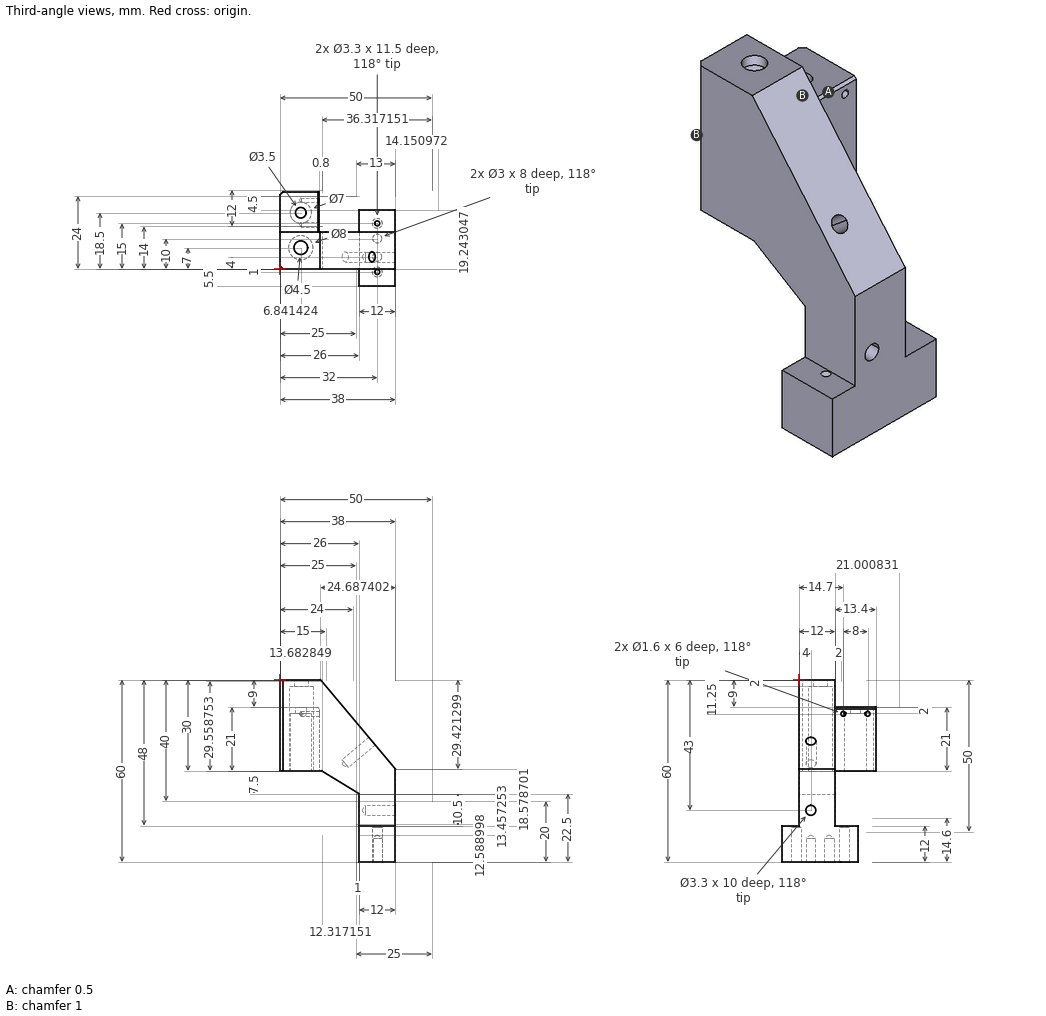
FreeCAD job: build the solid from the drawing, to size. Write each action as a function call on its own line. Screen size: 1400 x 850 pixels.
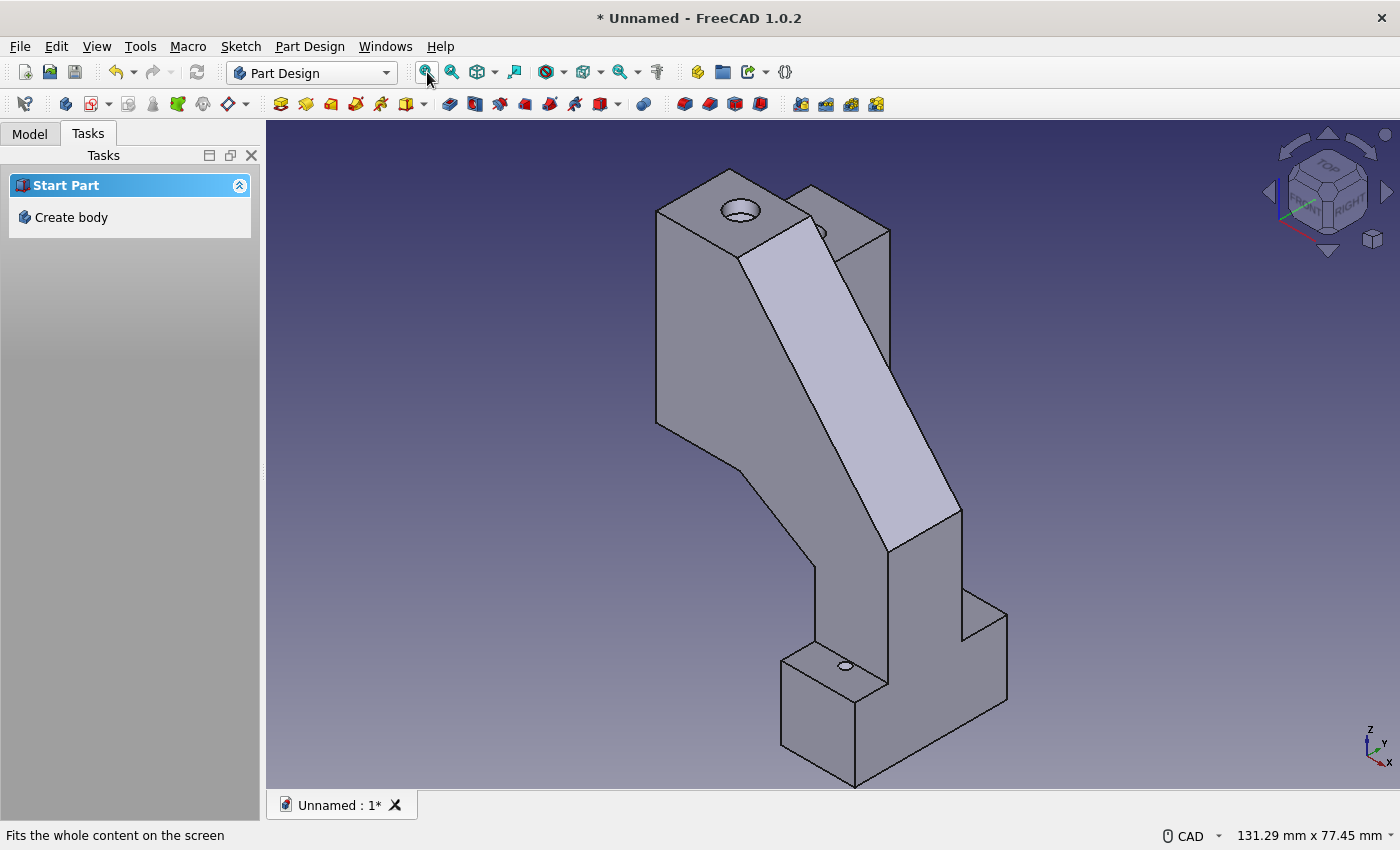
key(3)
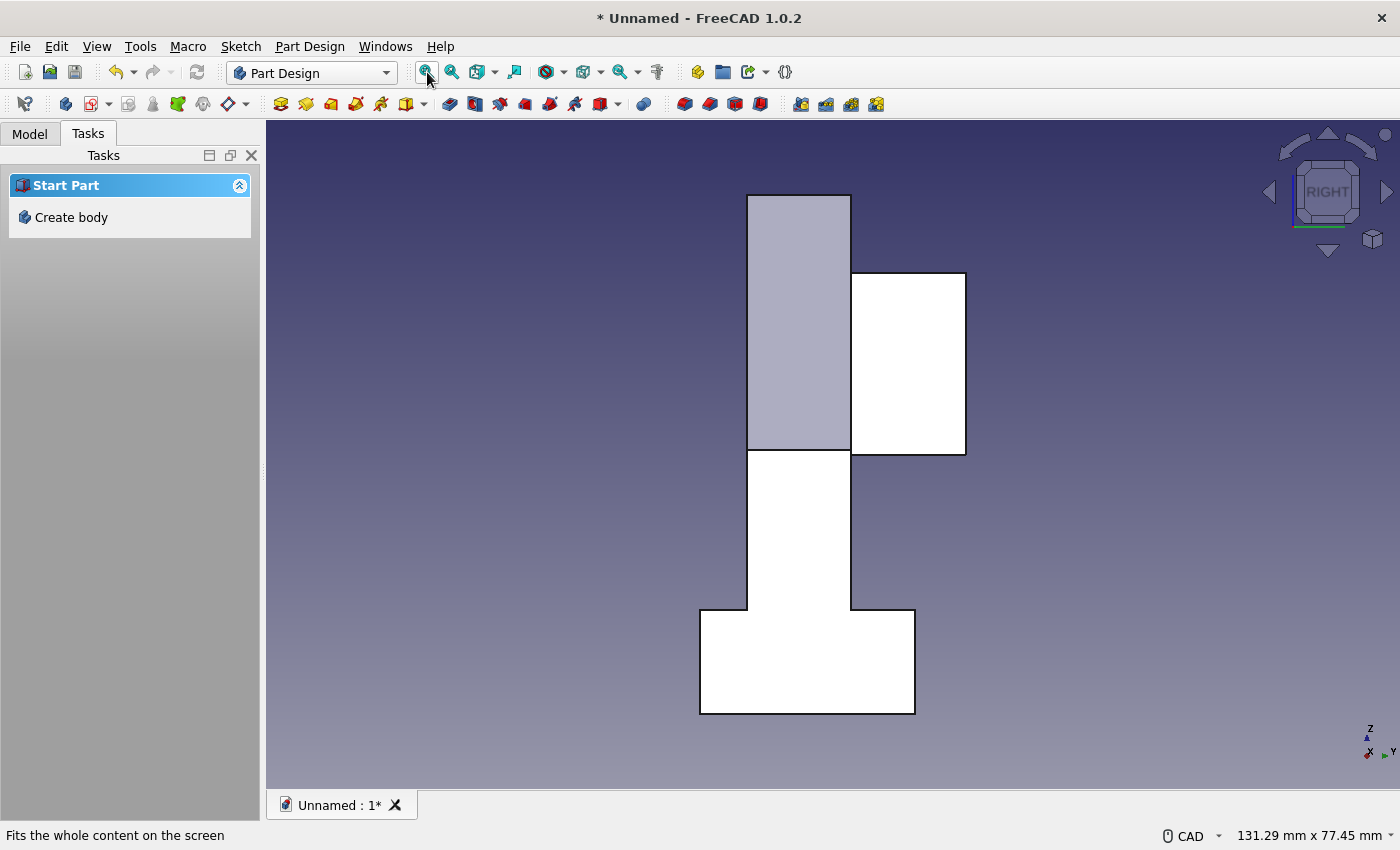
click(909, 337)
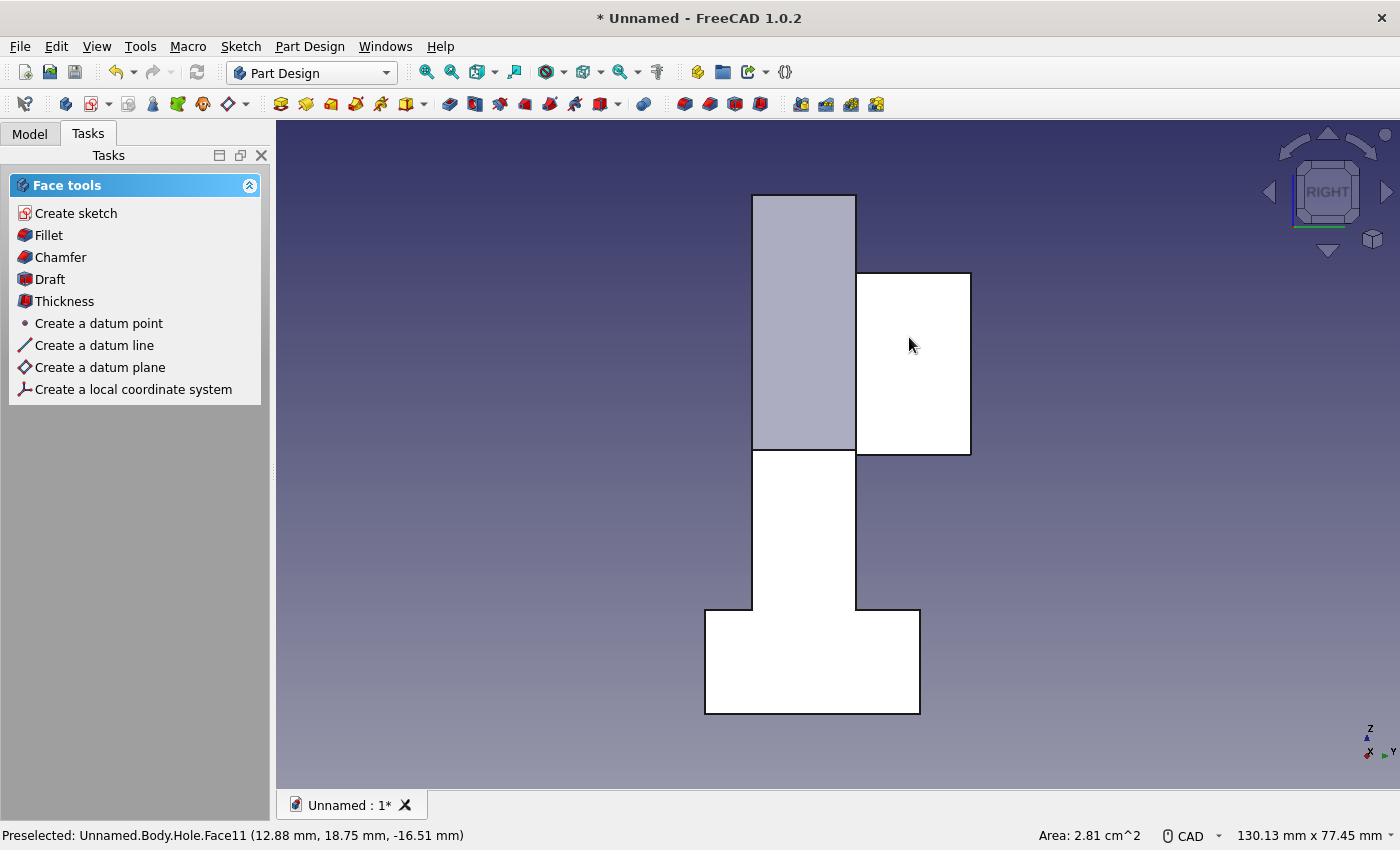
click(90, 104)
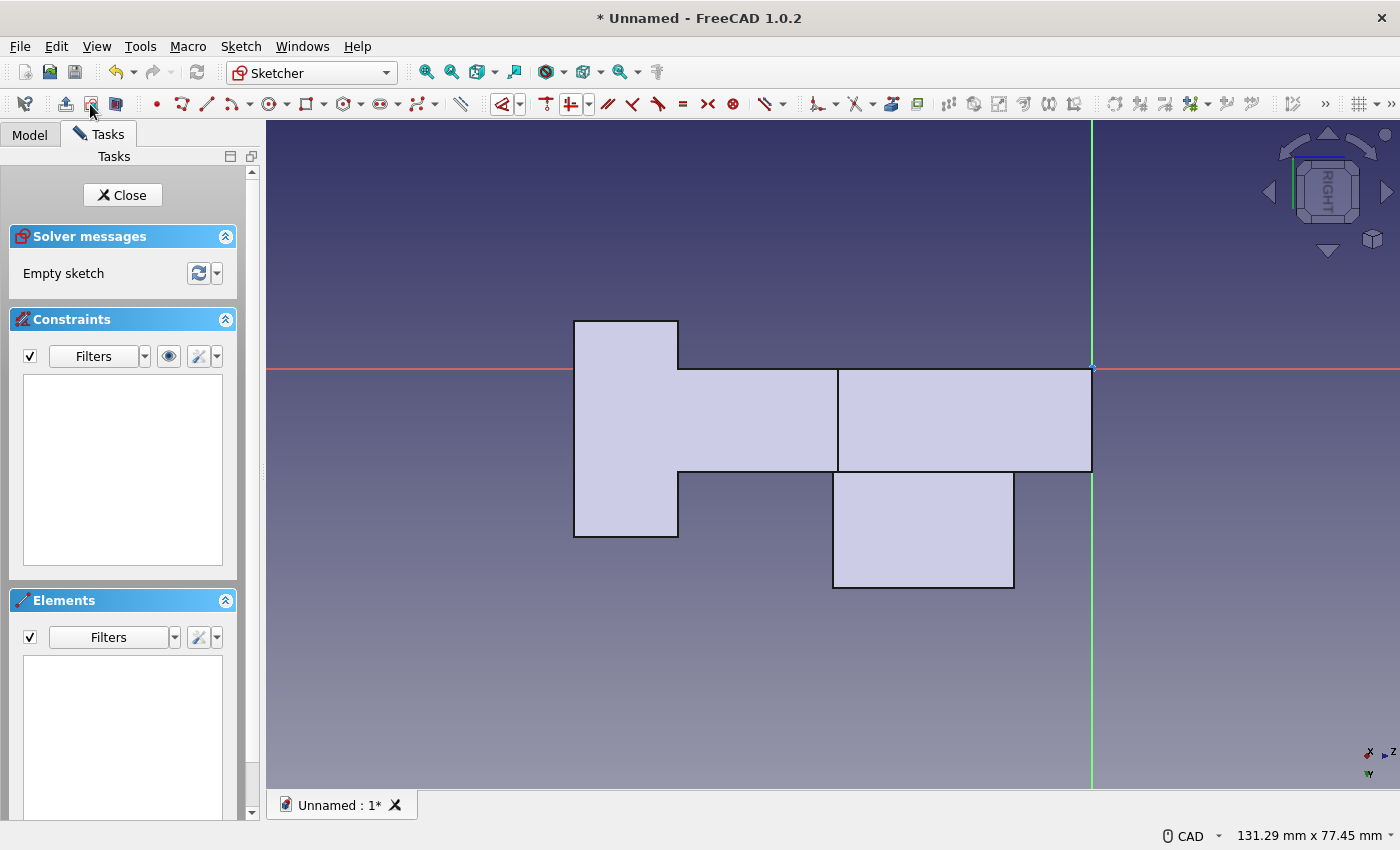
scroll(1235, 483, up, 4)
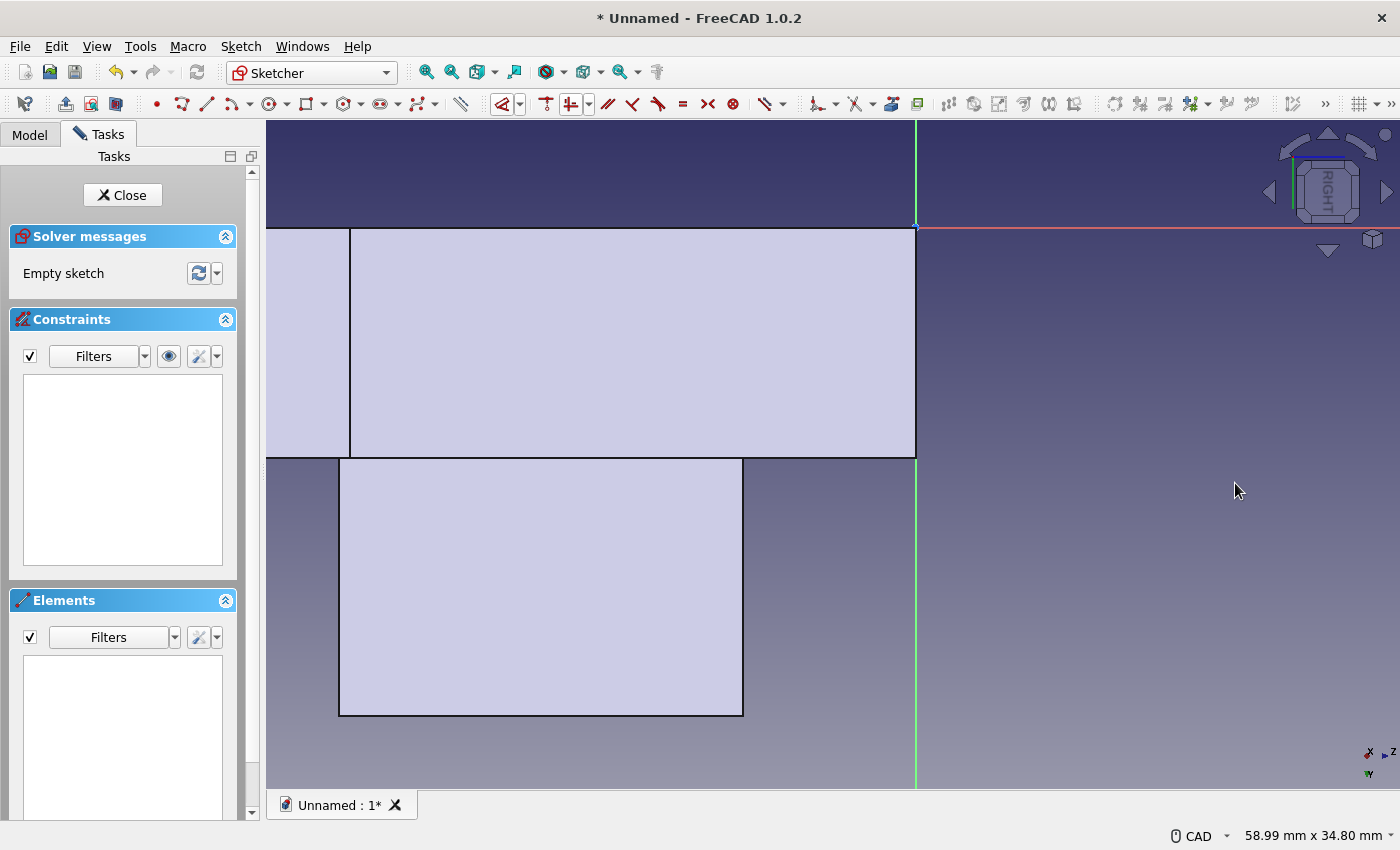
click(268, 104)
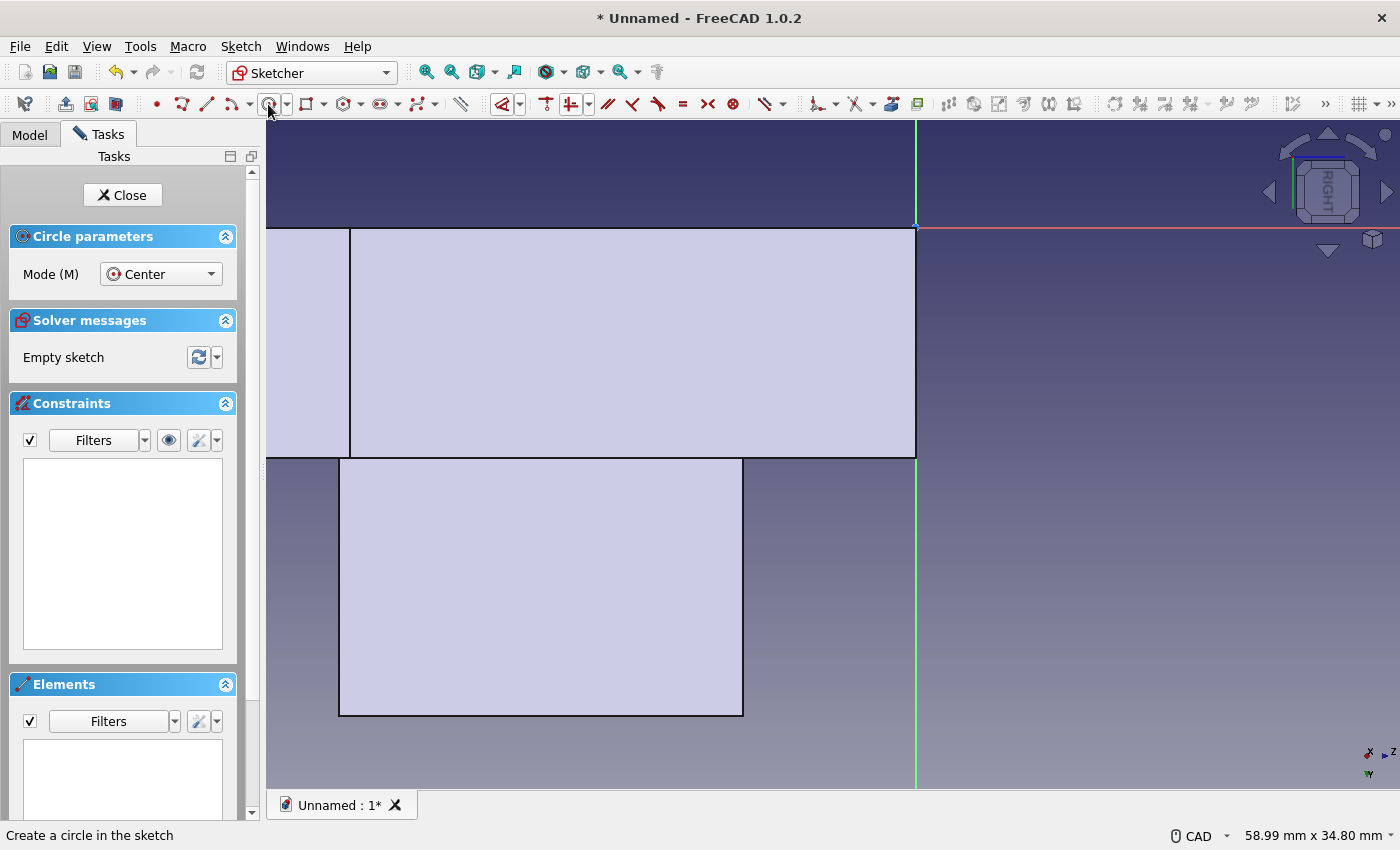
scroll(700, 510, up, 2)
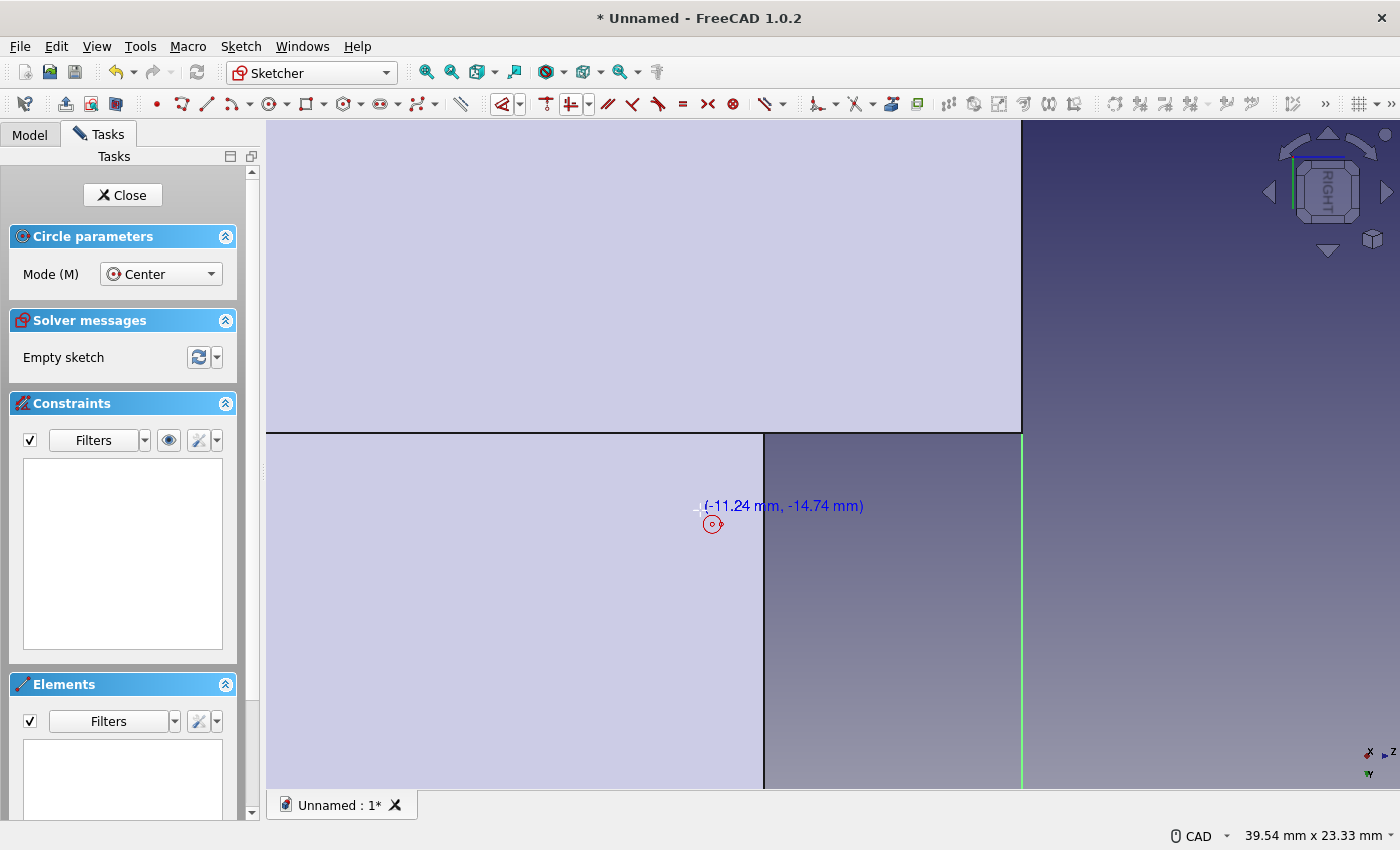
click(699, 510)
click(716, 494)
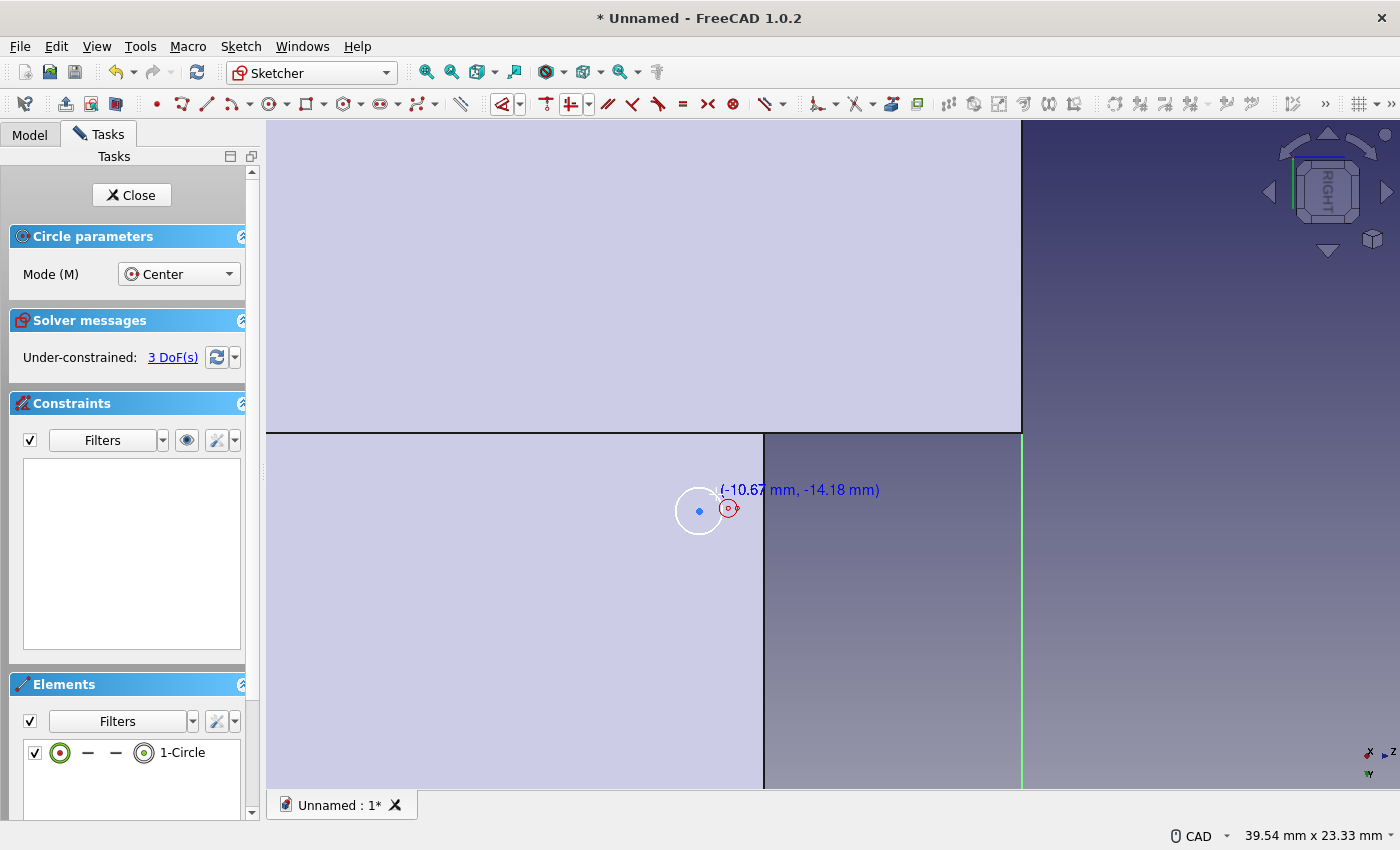
click(699, 739)
click(716, 723)
key(Escape)